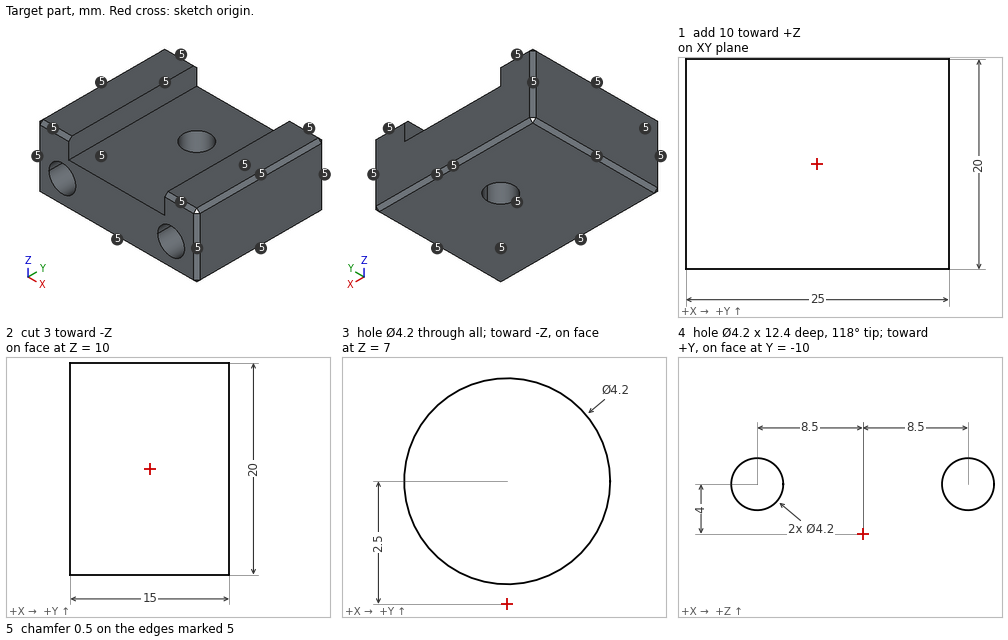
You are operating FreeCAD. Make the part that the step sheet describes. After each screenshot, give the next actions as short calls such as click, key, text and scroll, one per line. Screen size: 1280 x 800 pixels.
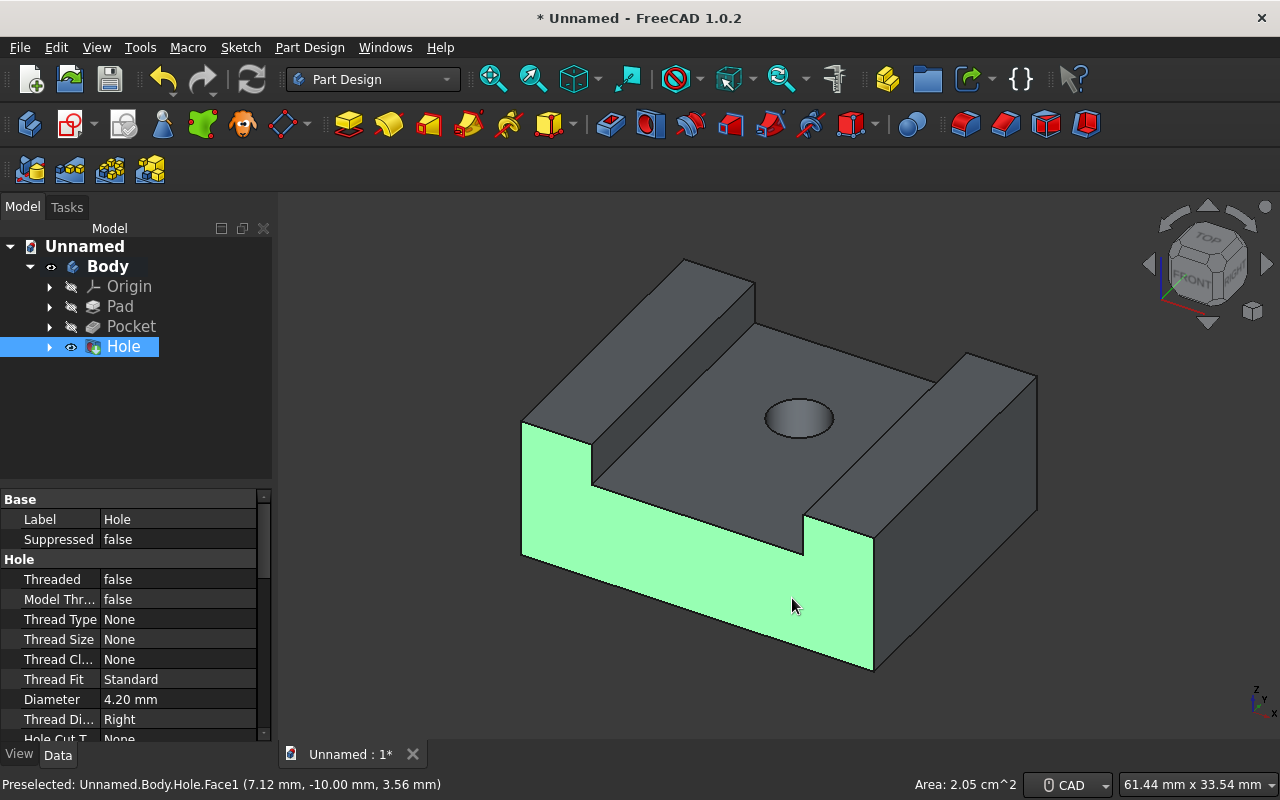
click(70, 124)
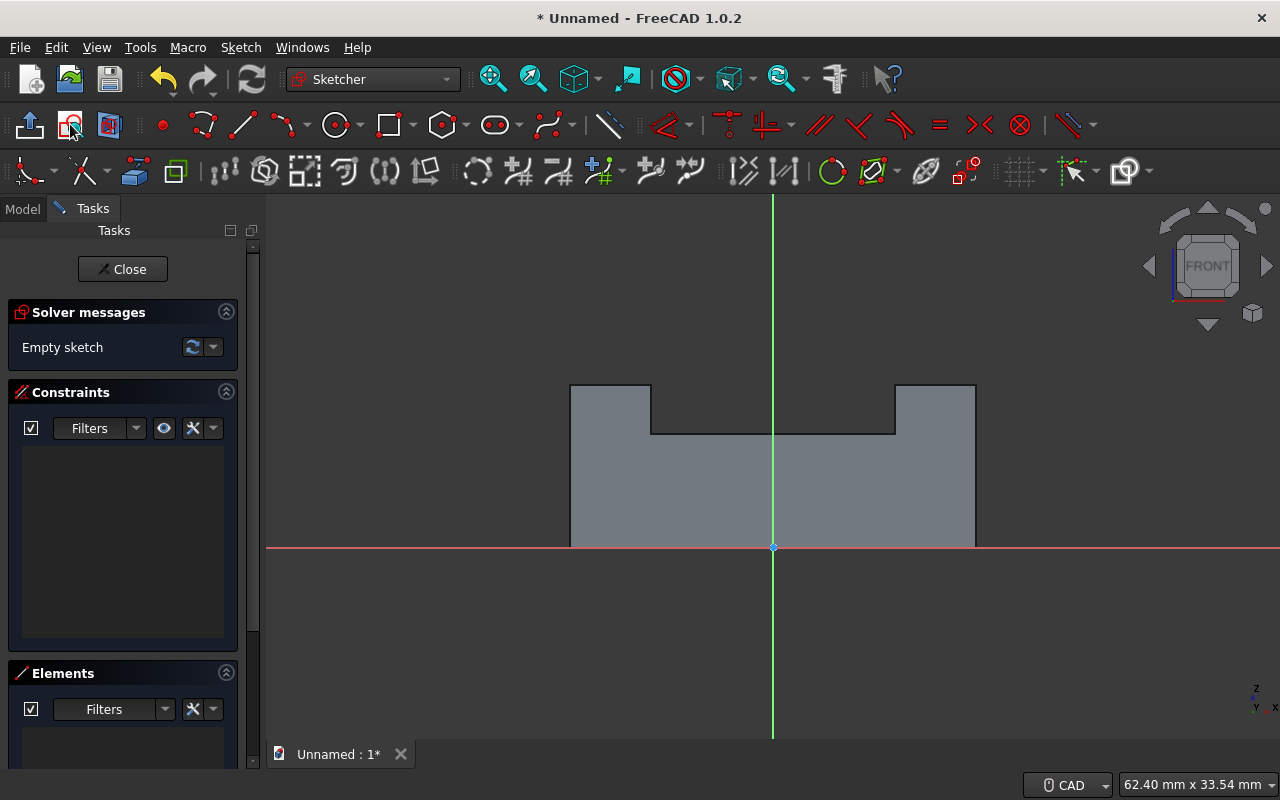
scroll(856, 537, up, 3)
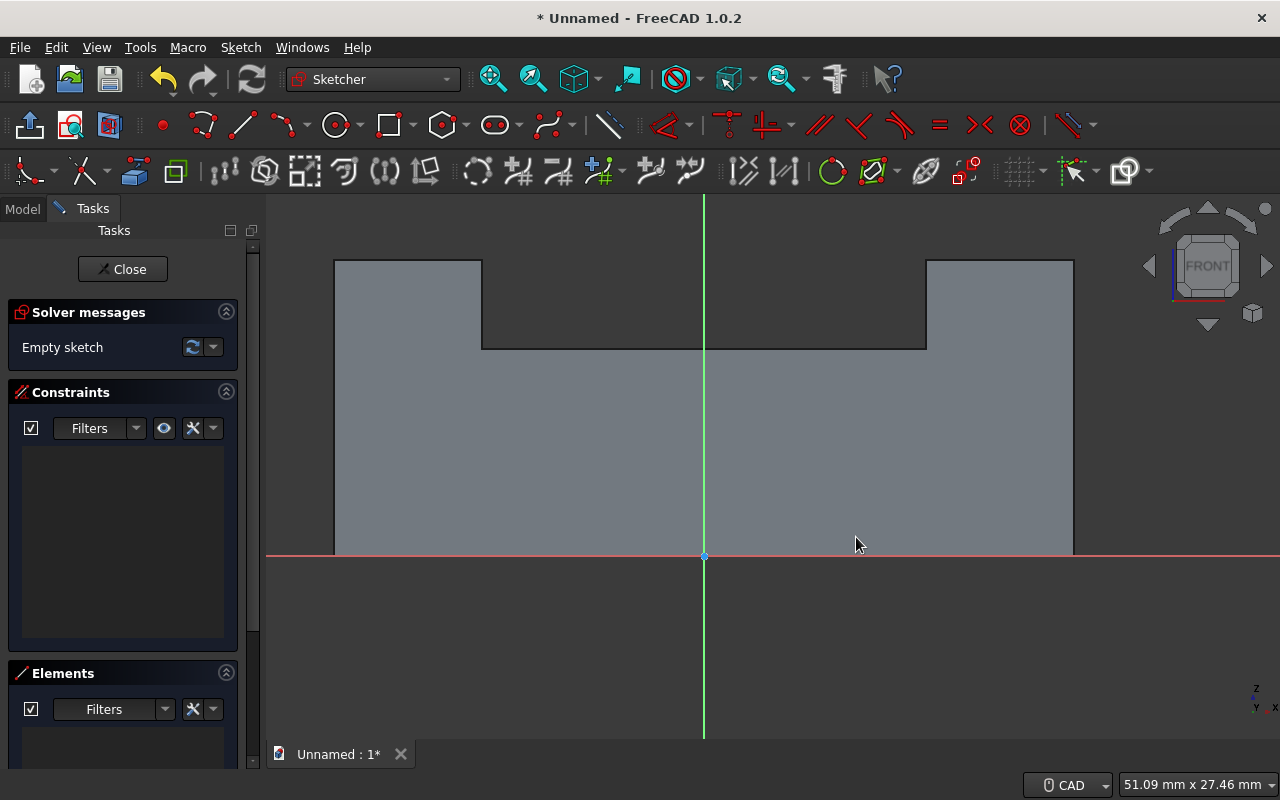
key(g)
key(c)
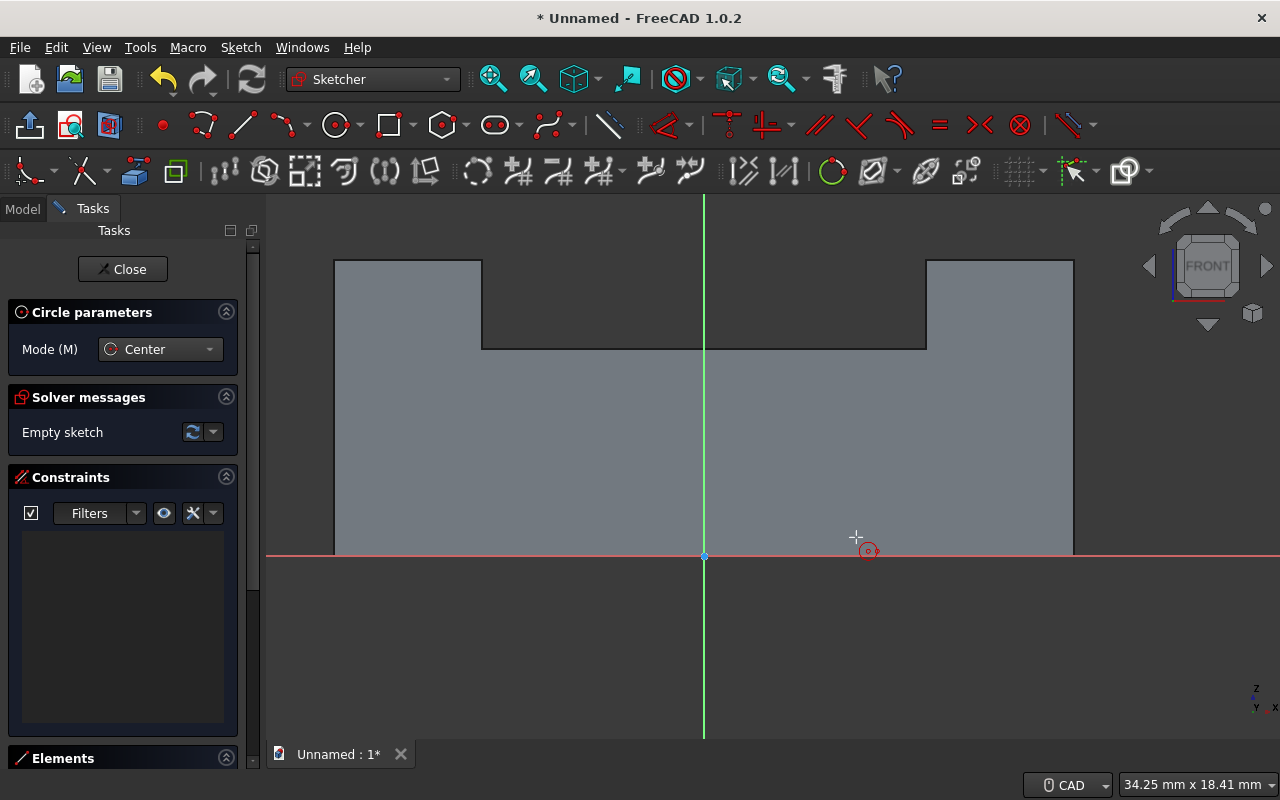
click(453, 438)
move(497, 394)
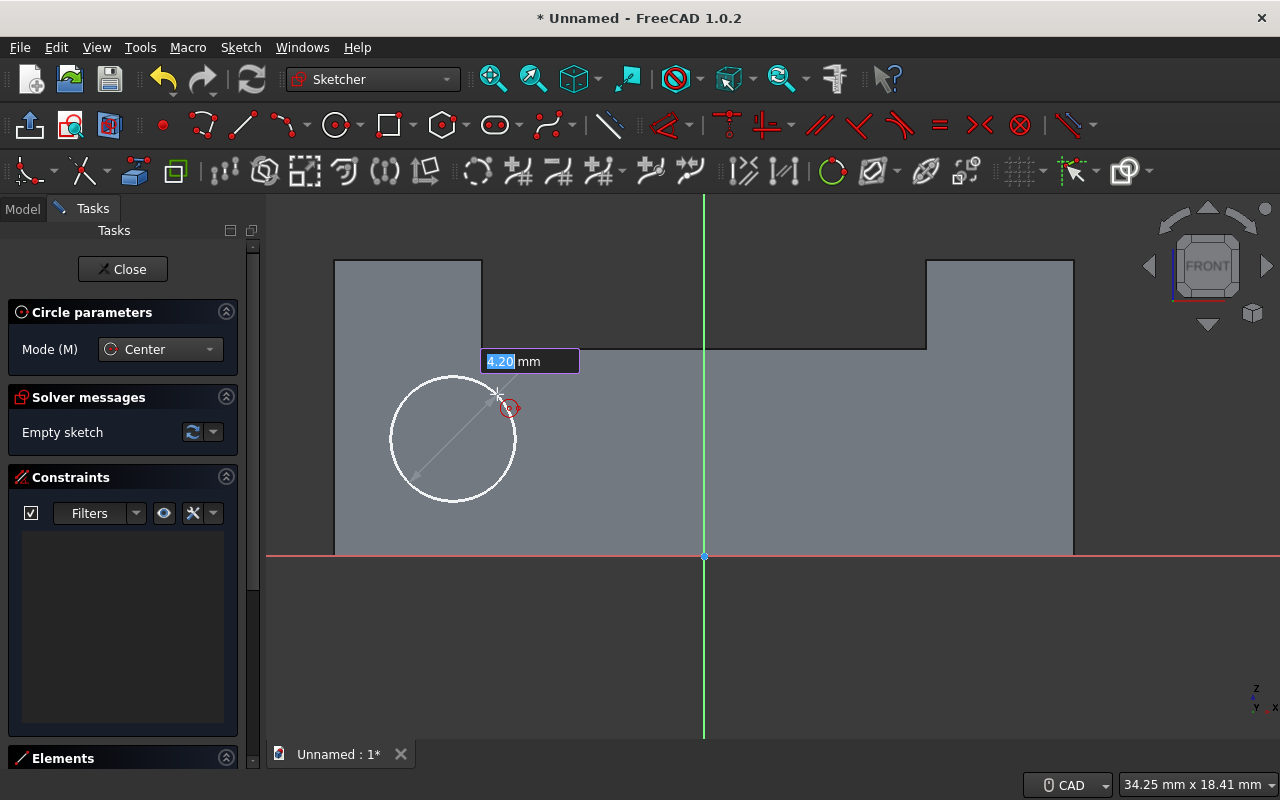
text(4.2)
key(Return)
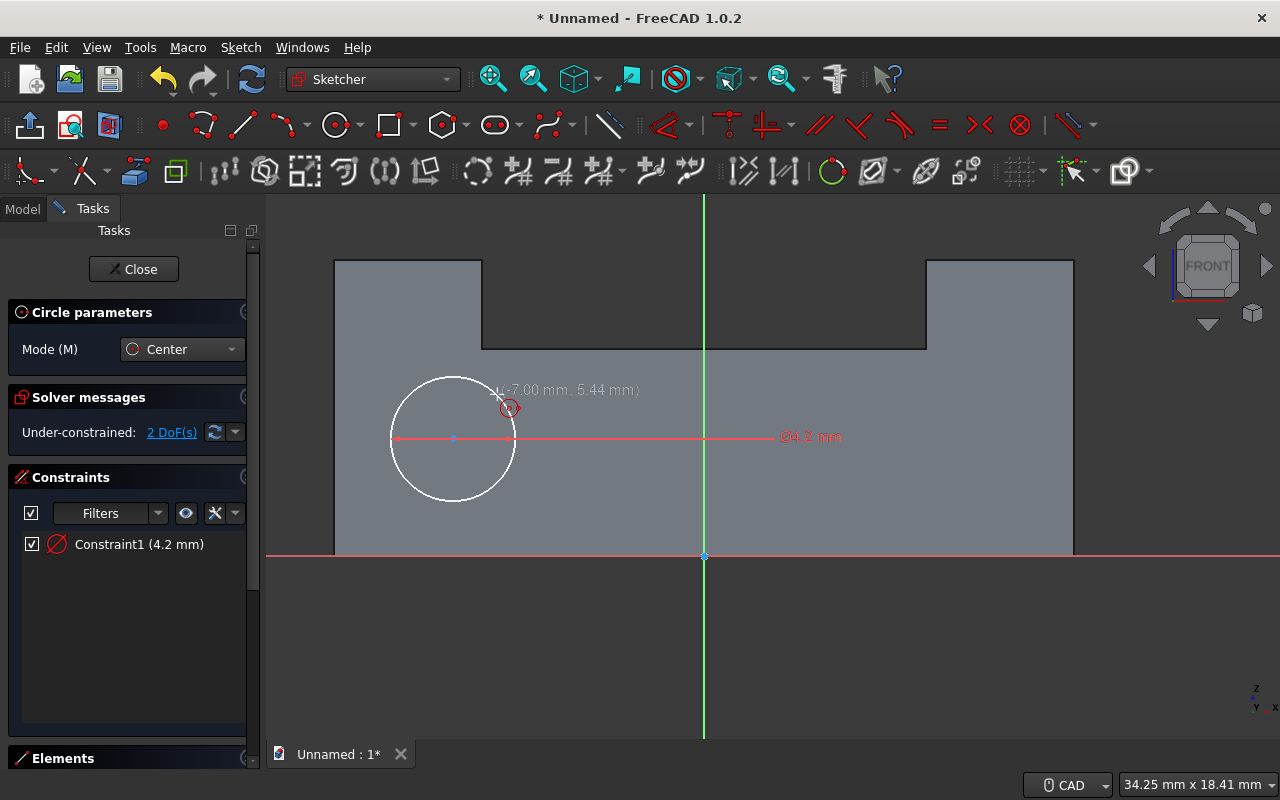
click(956, 438)
move(1000, 394)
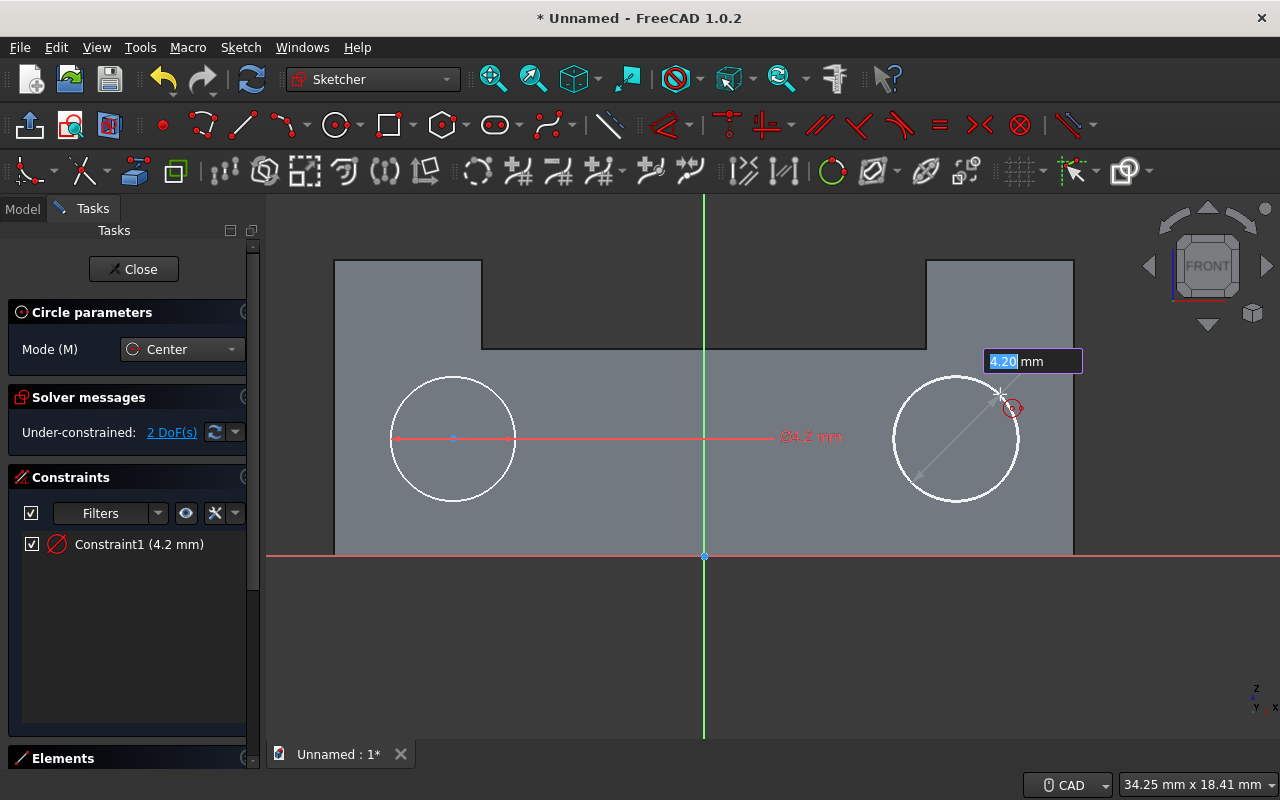
text(4.2)
key(Return)
key(Escape)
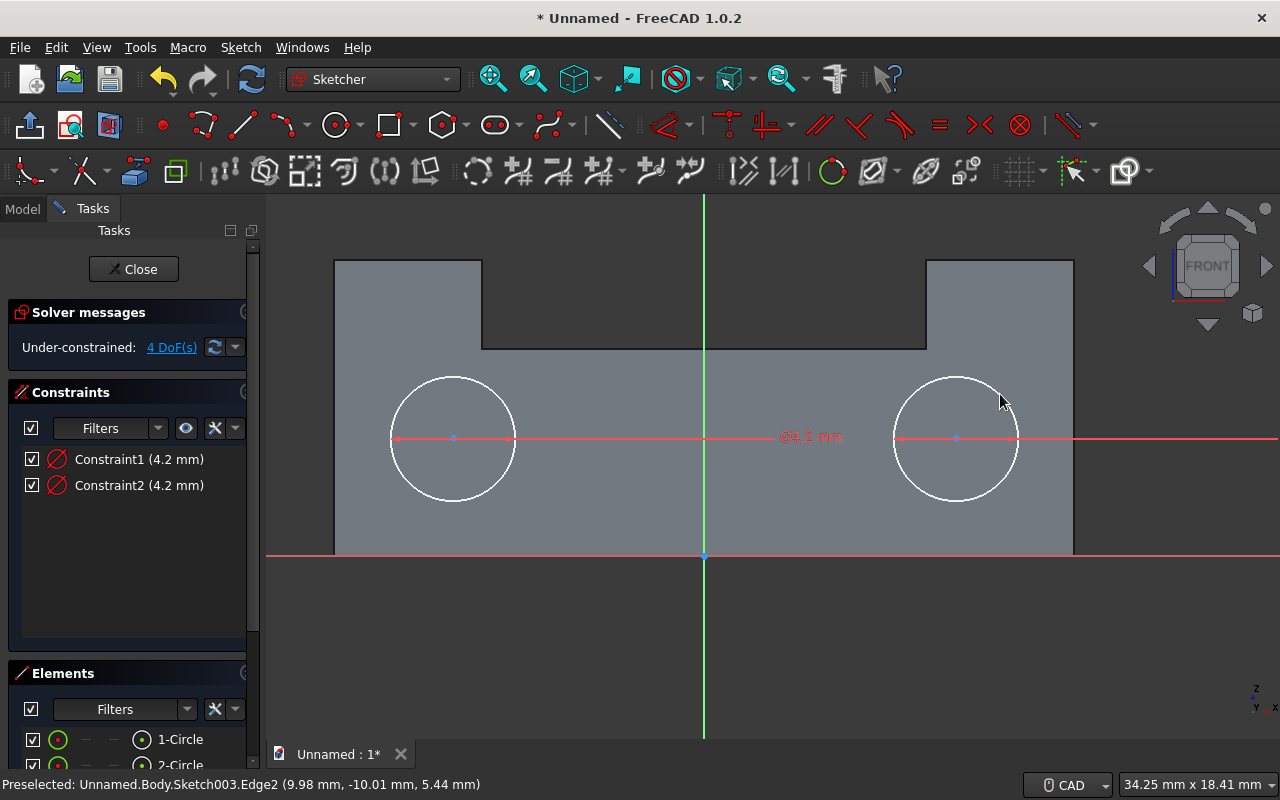
click(453, 439)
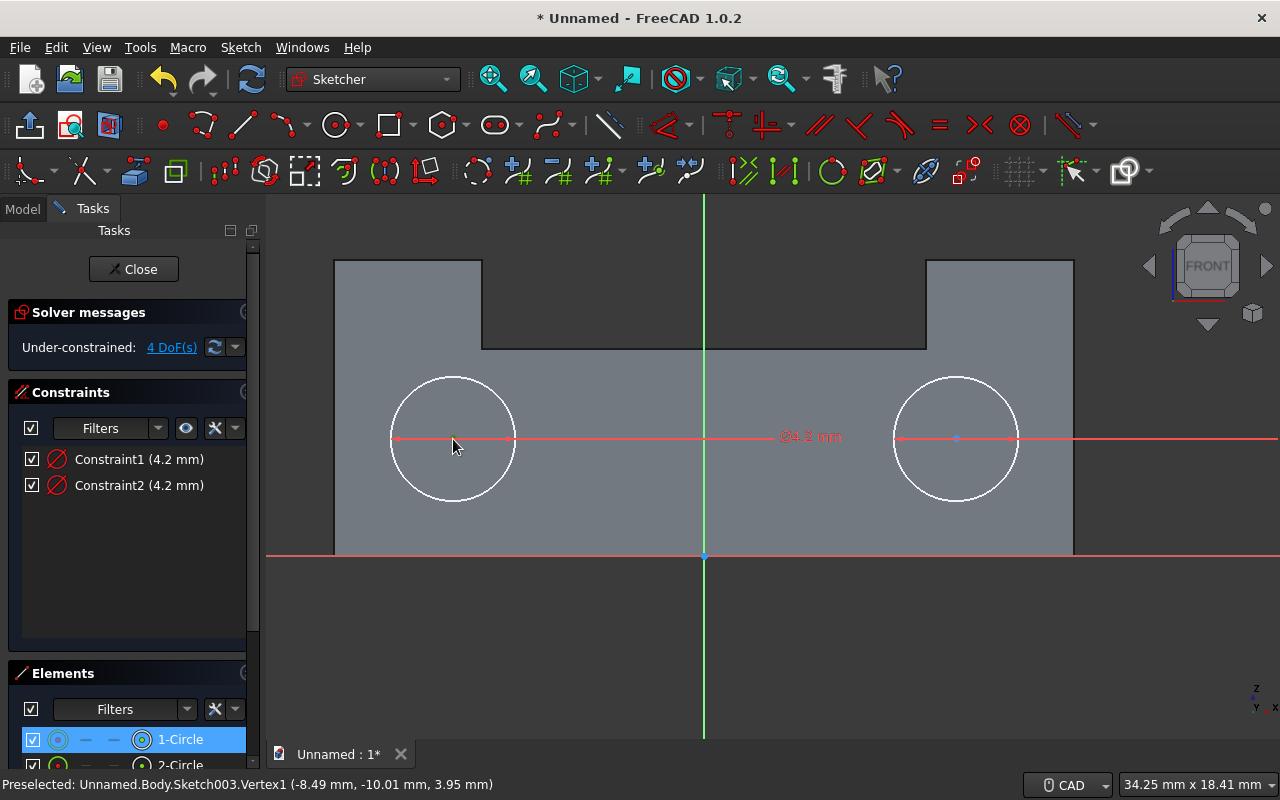
click(956, 439)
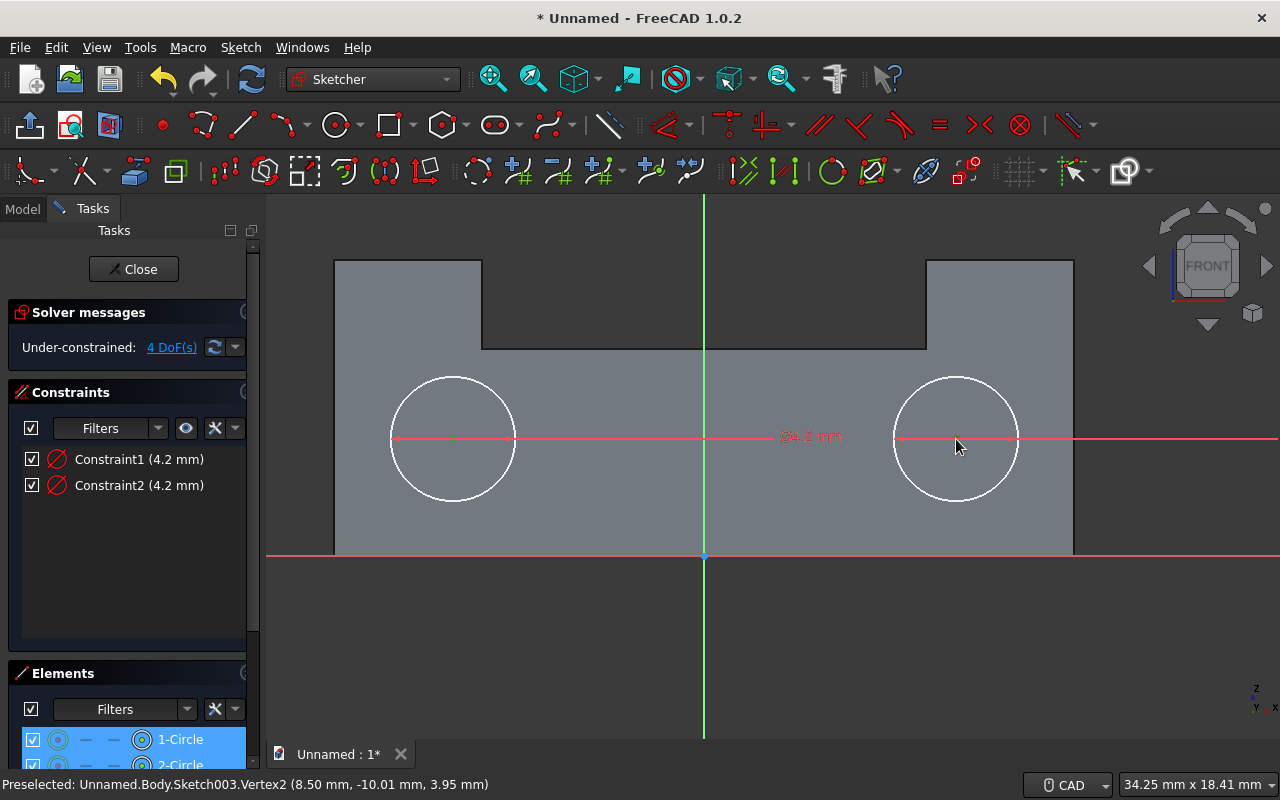
click(794, 126)